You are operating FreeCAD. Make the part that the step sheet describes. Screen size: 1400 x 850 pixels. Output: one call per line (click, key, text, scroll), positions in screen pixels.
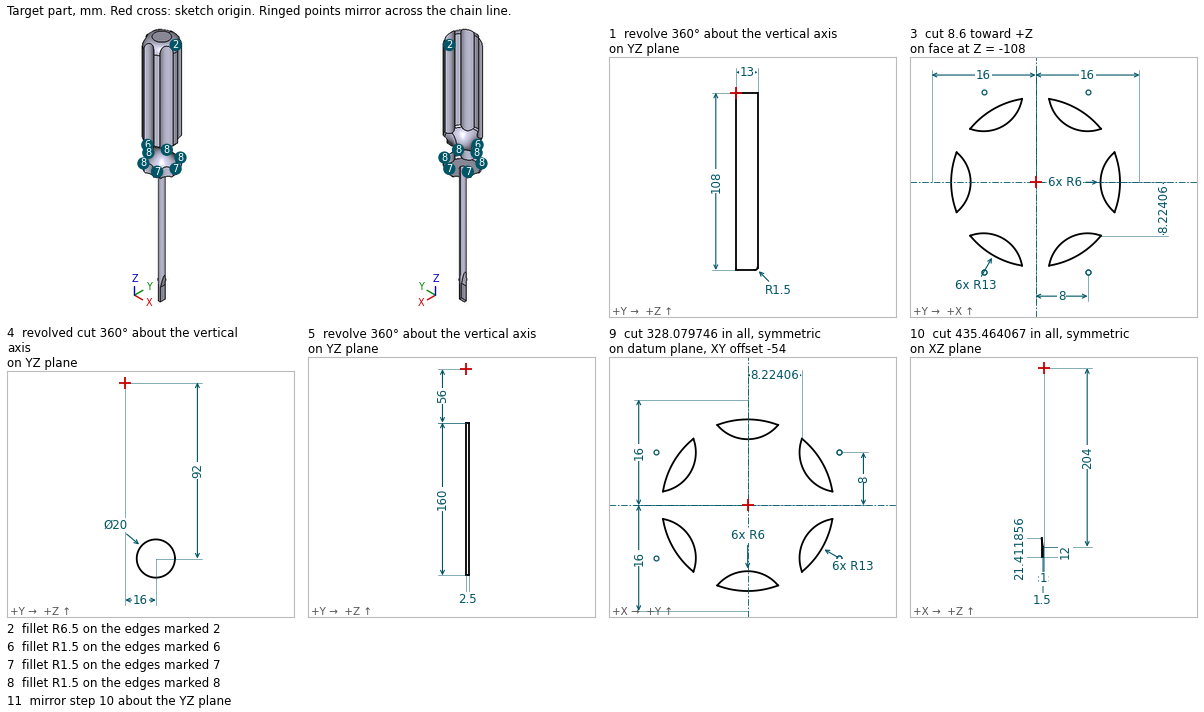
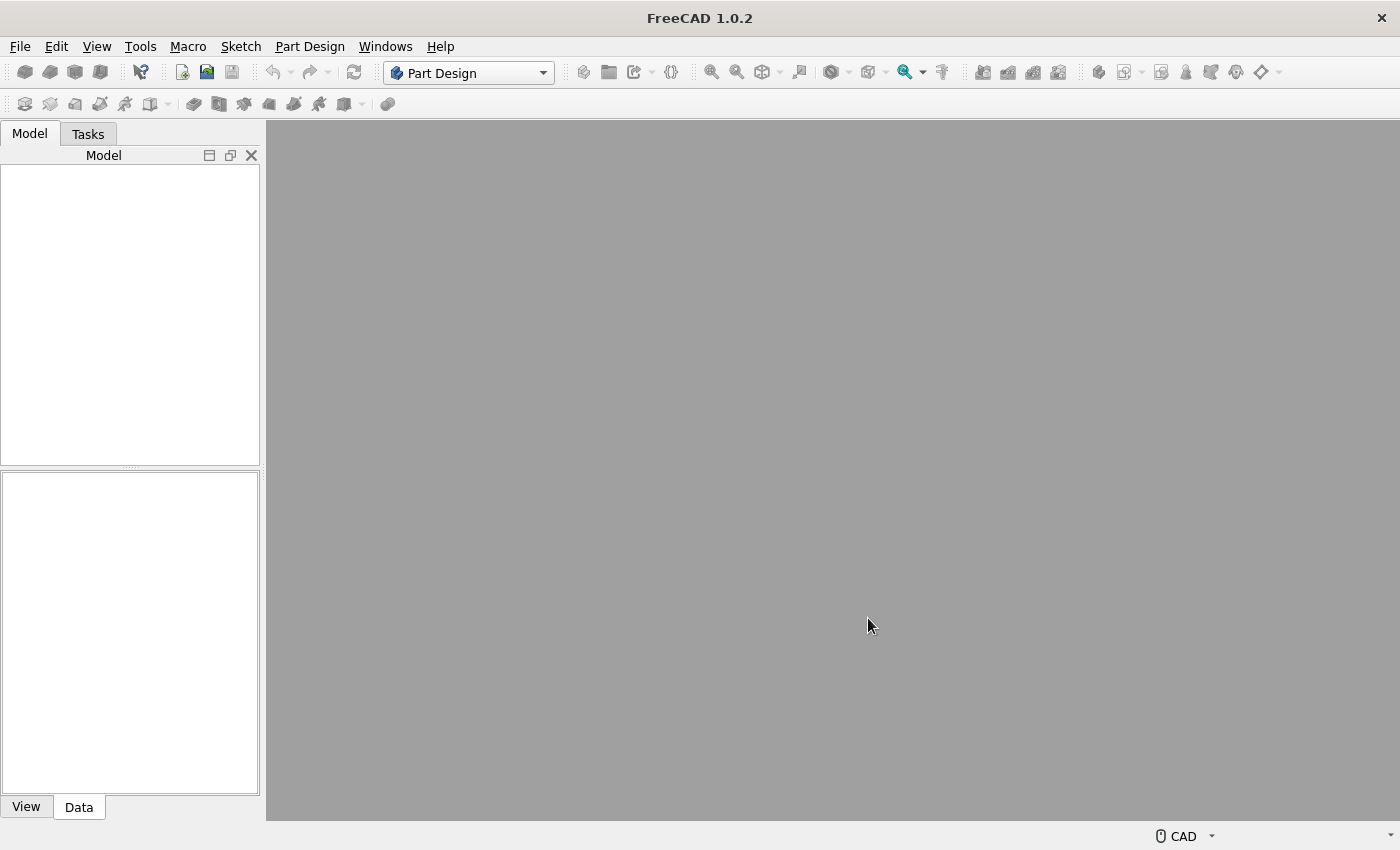
key(ctrl+n)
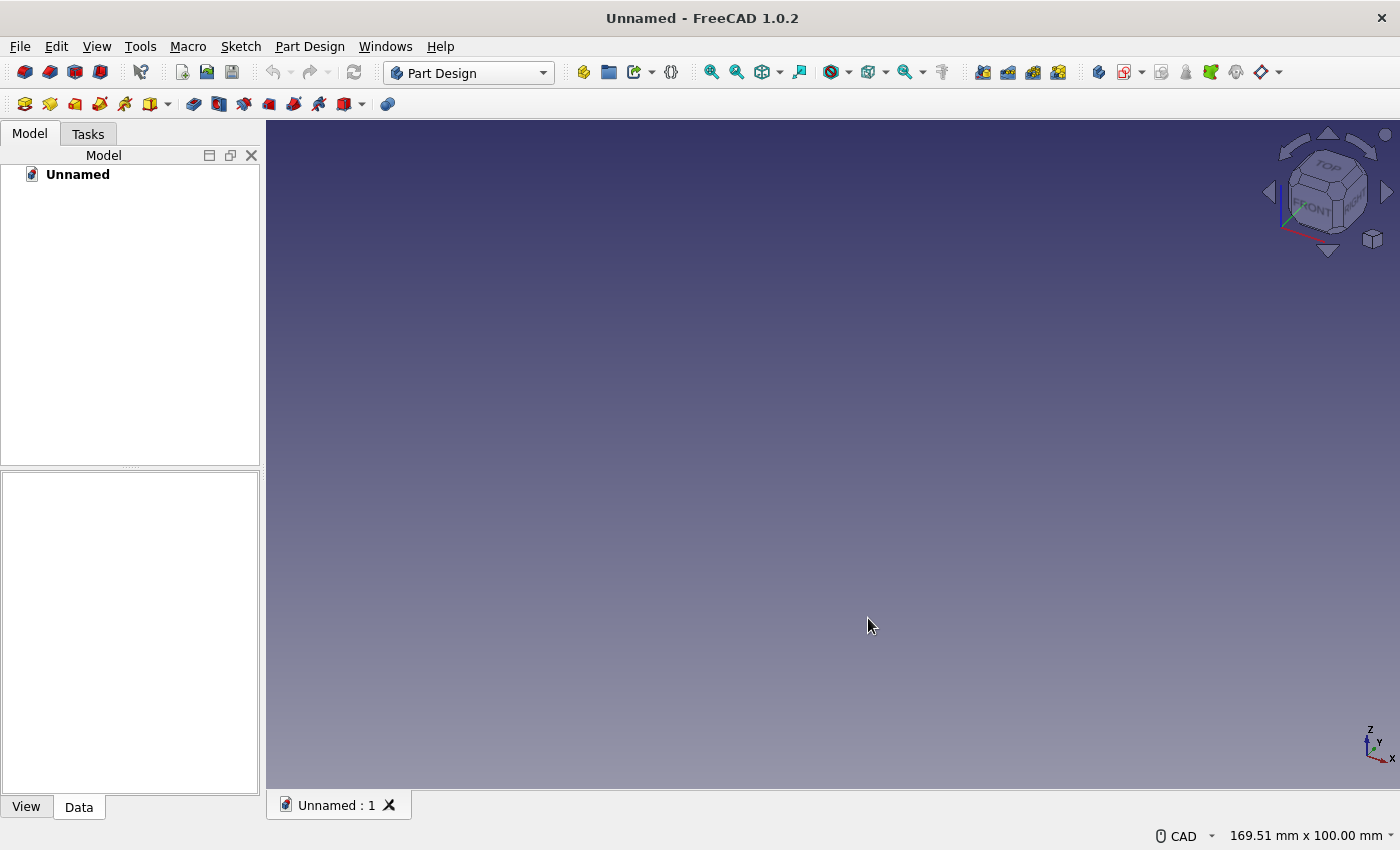
click(1124, 72)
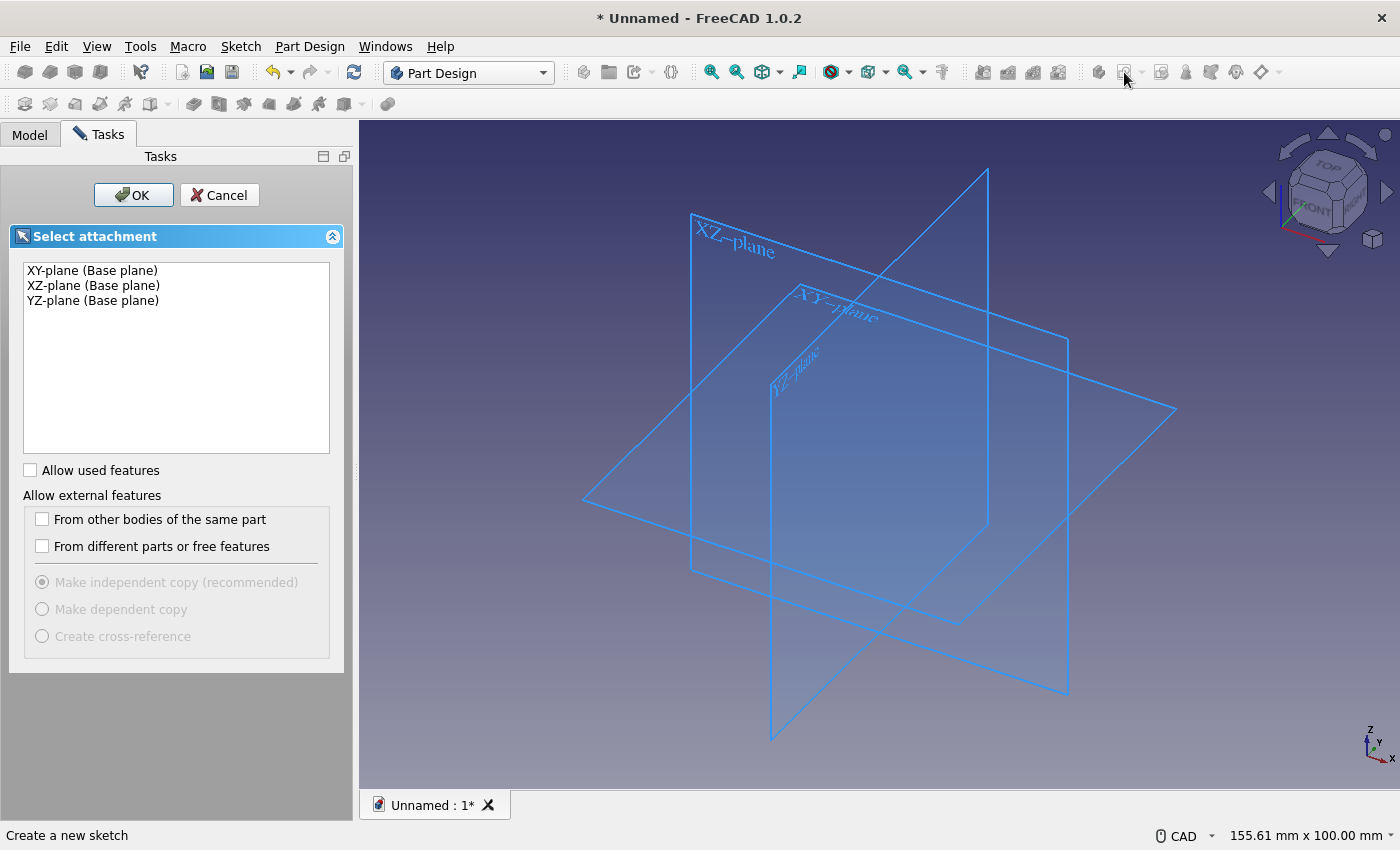
click(84, 300)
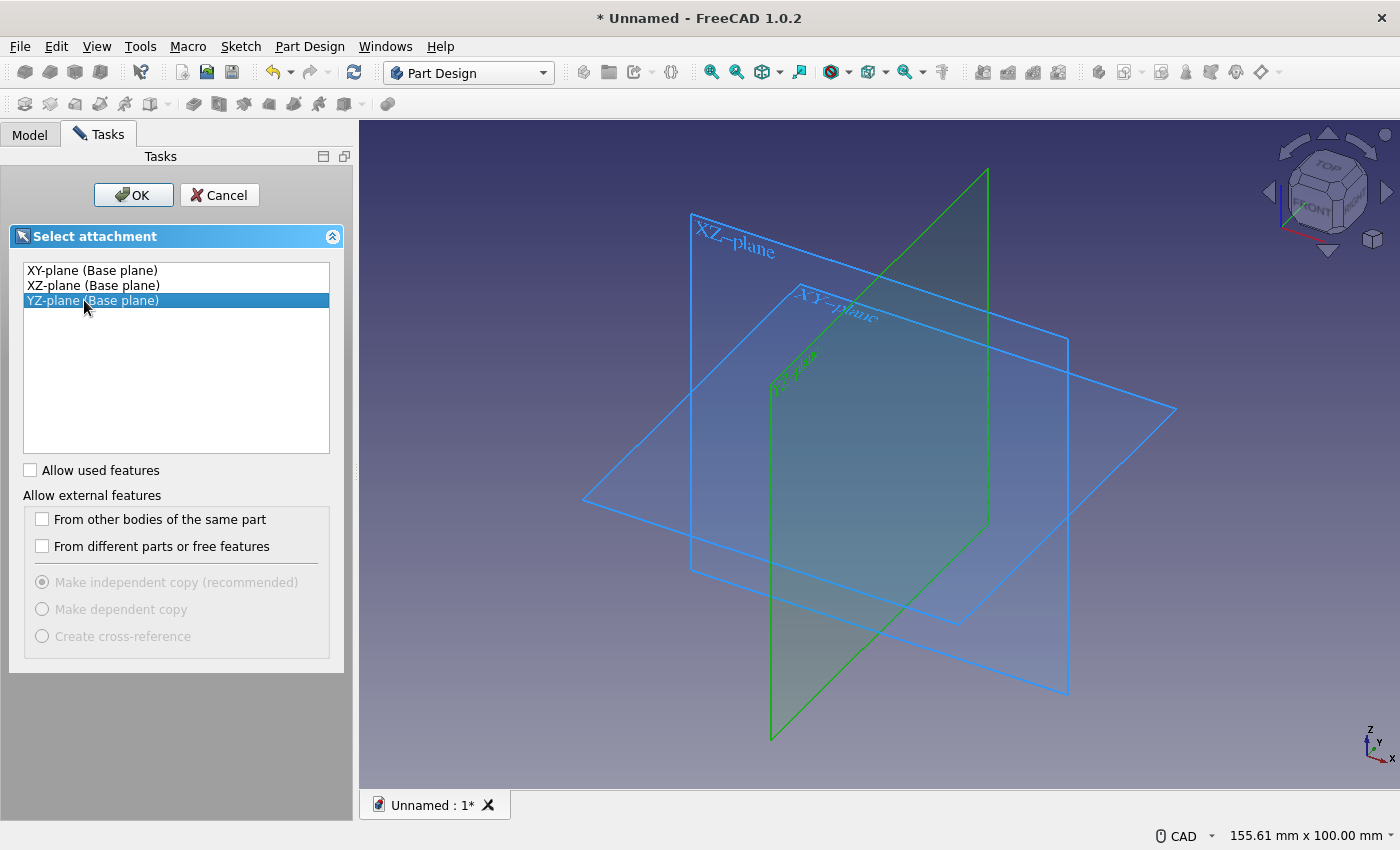
click(134, 195)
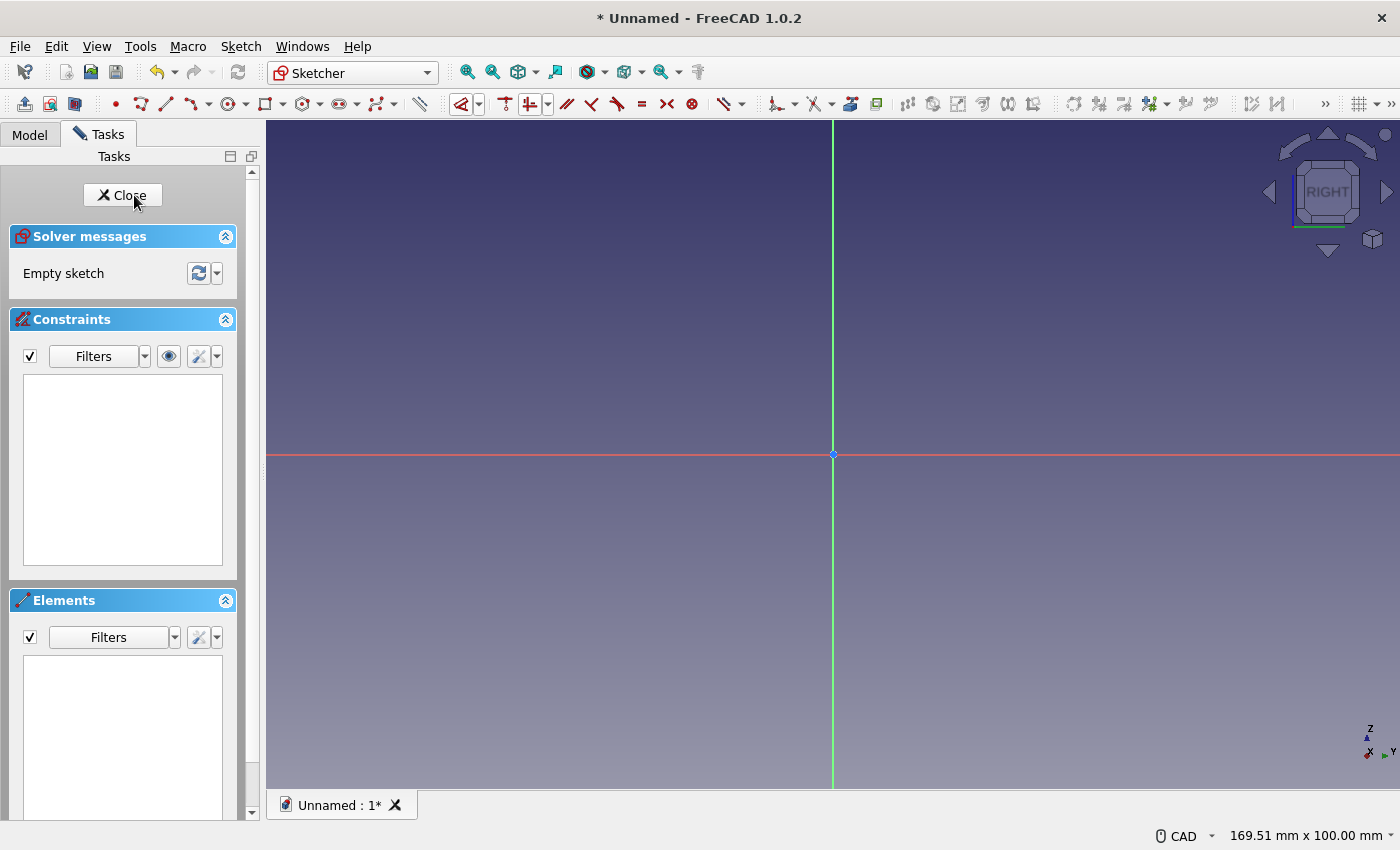
scroll(628, 148, down, 3)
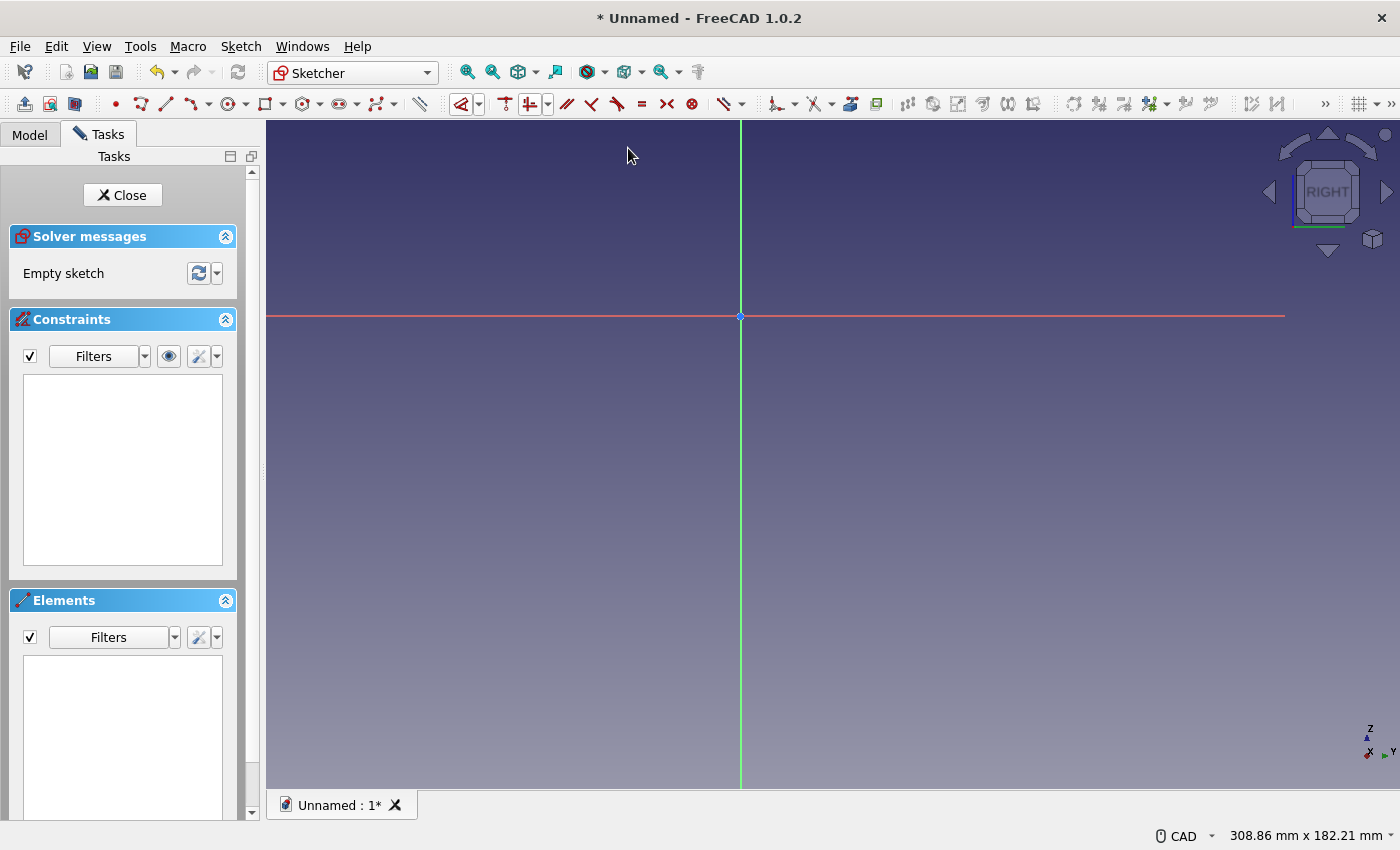
click(141, 104)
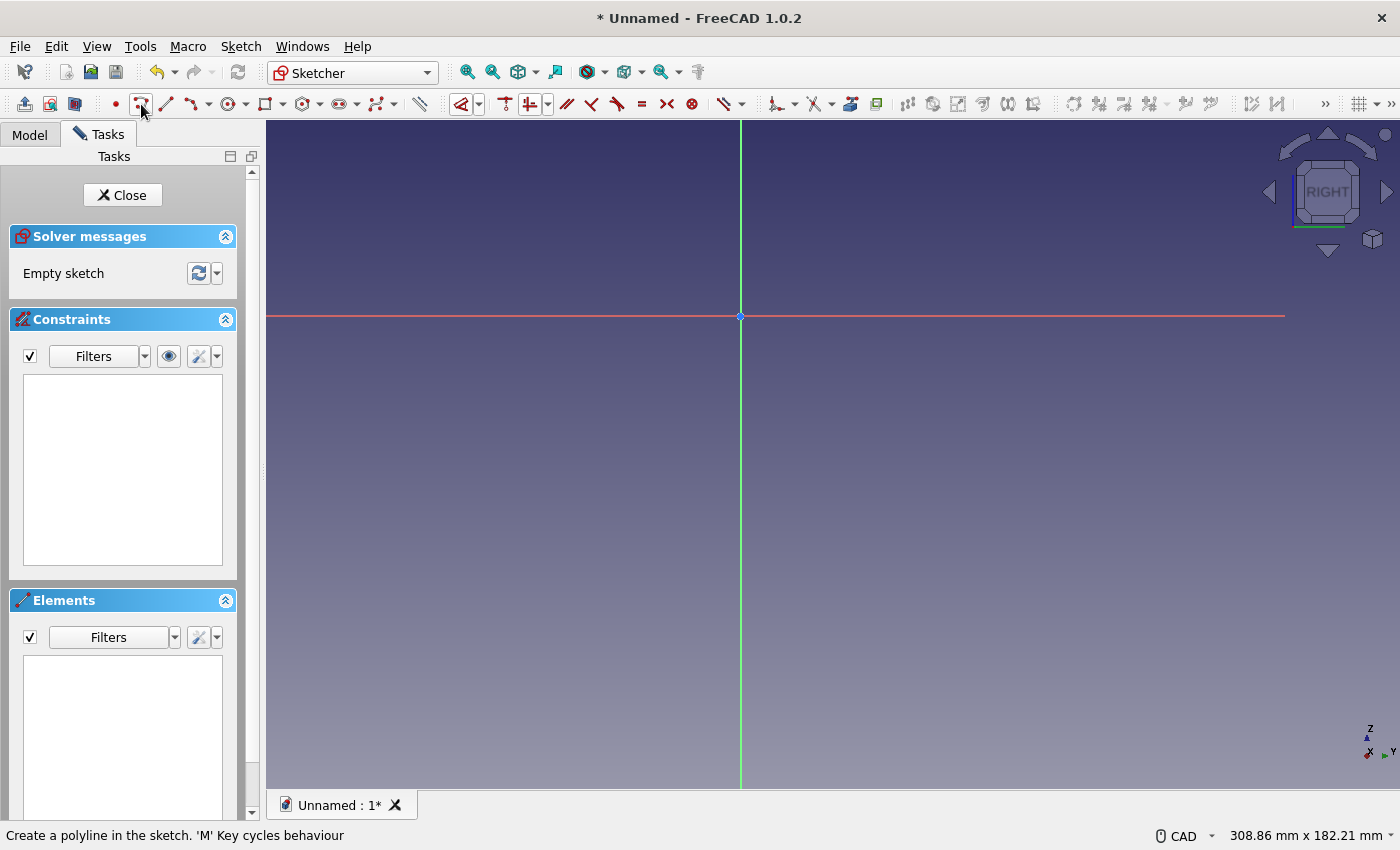
click(788, 707)
click(788, 316)
click(741, 316)
click(750, 713)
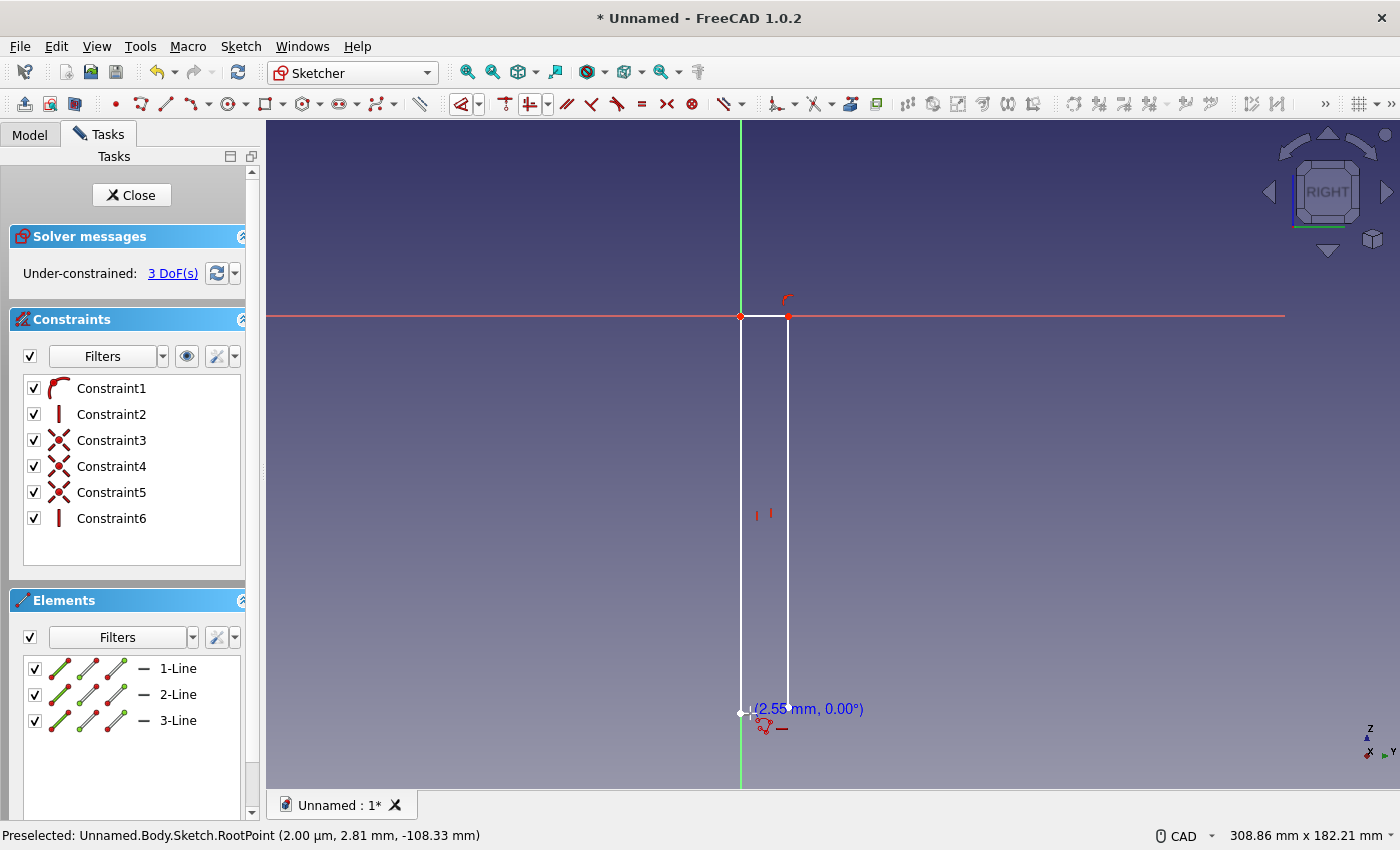
scroll(783, 713, up, 4)